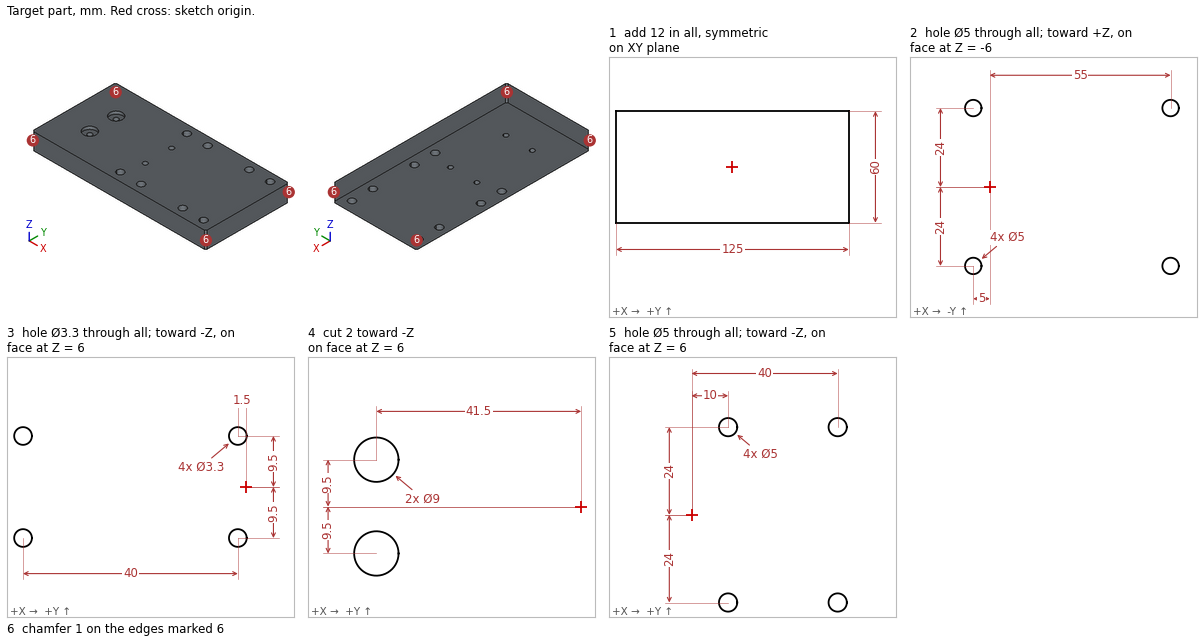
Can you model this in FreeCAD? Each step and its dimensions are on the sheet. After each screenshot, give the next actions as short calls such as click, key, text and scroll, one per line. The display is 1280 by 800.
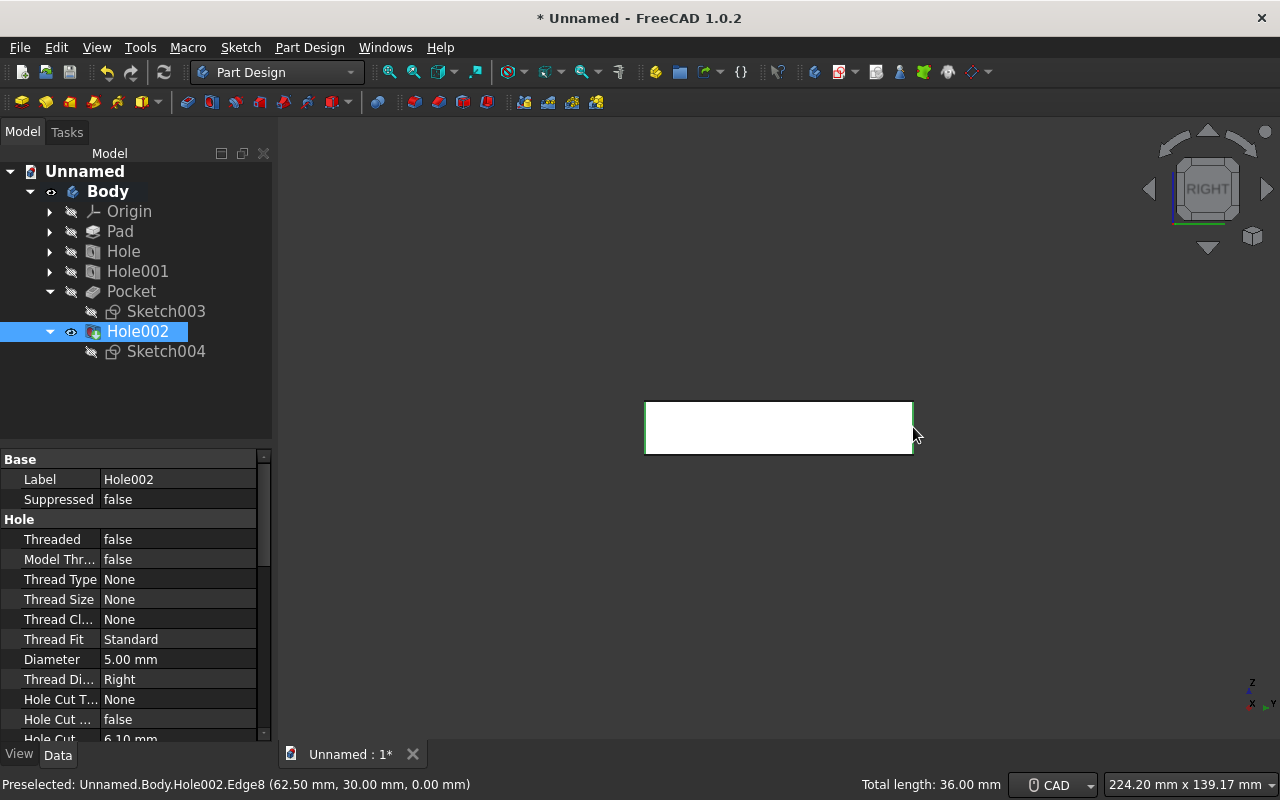
key(5)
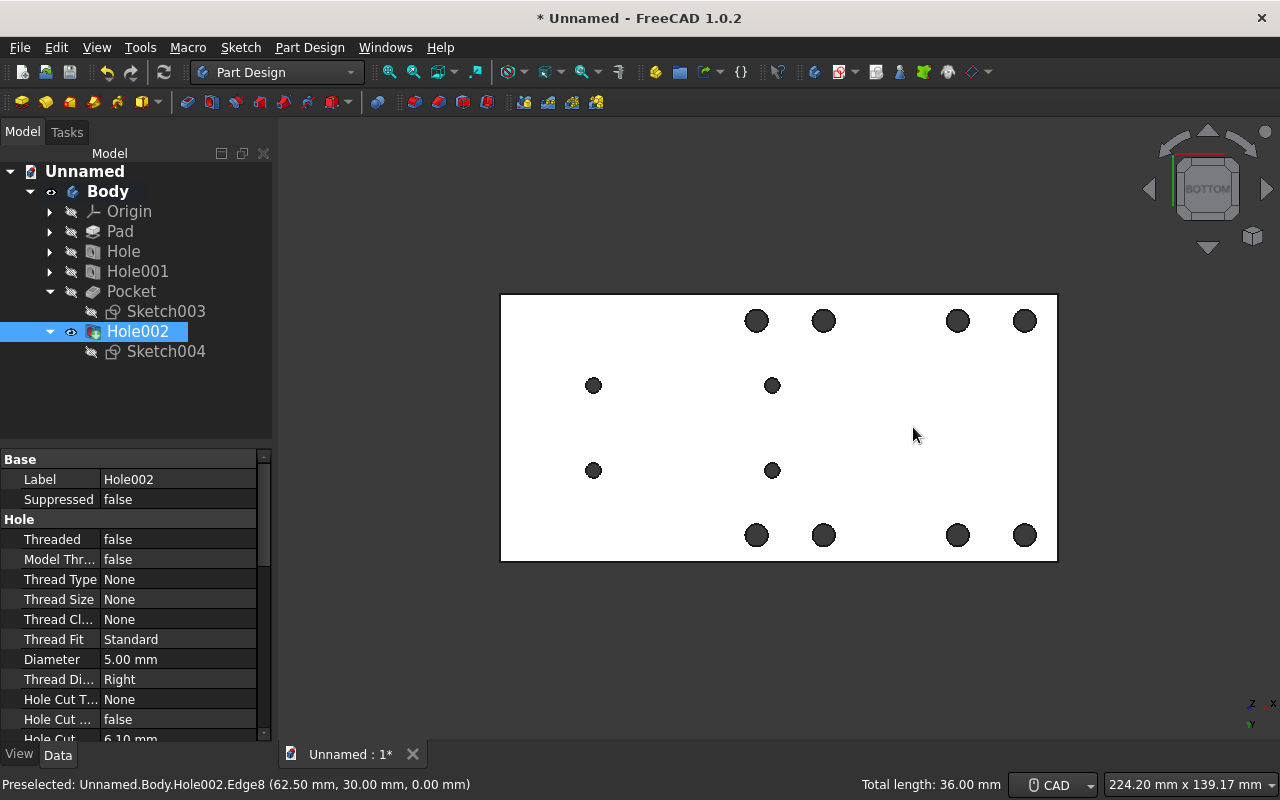
key(4)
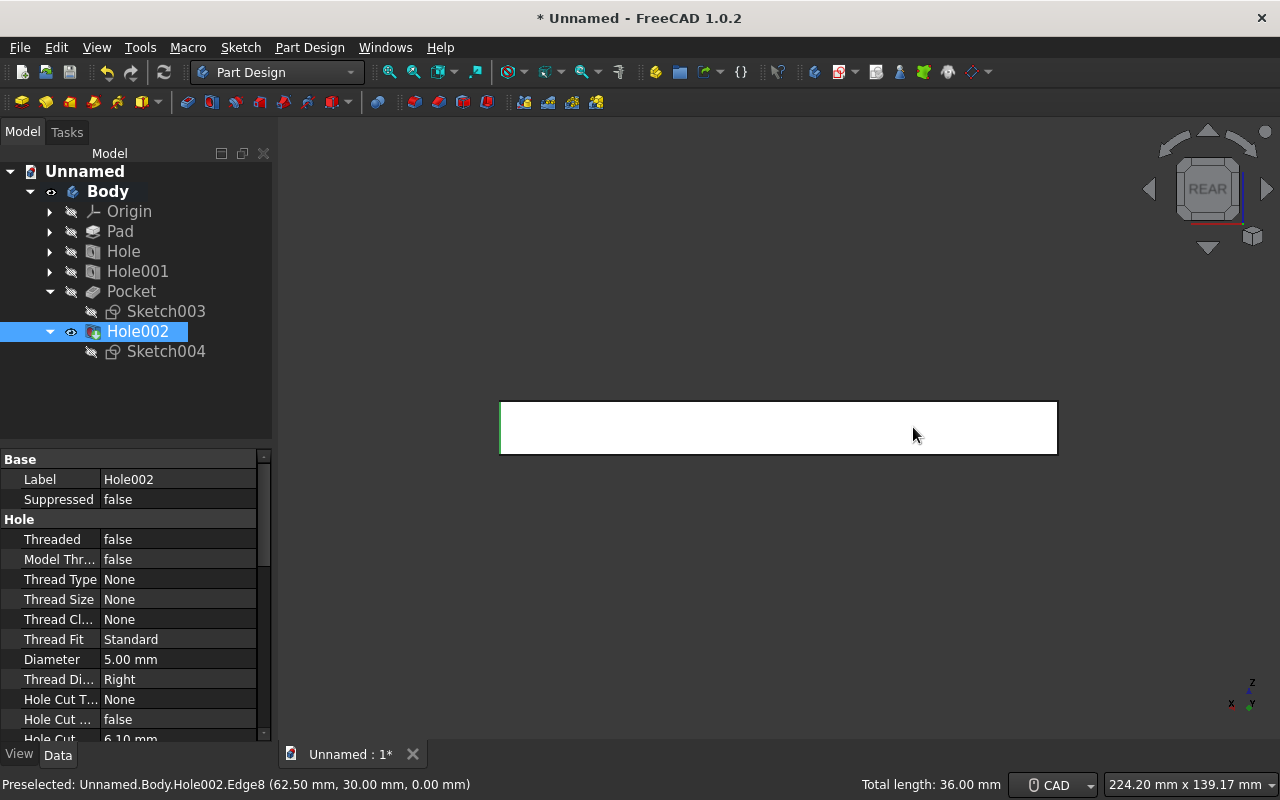
click(1058, 427, ctrl)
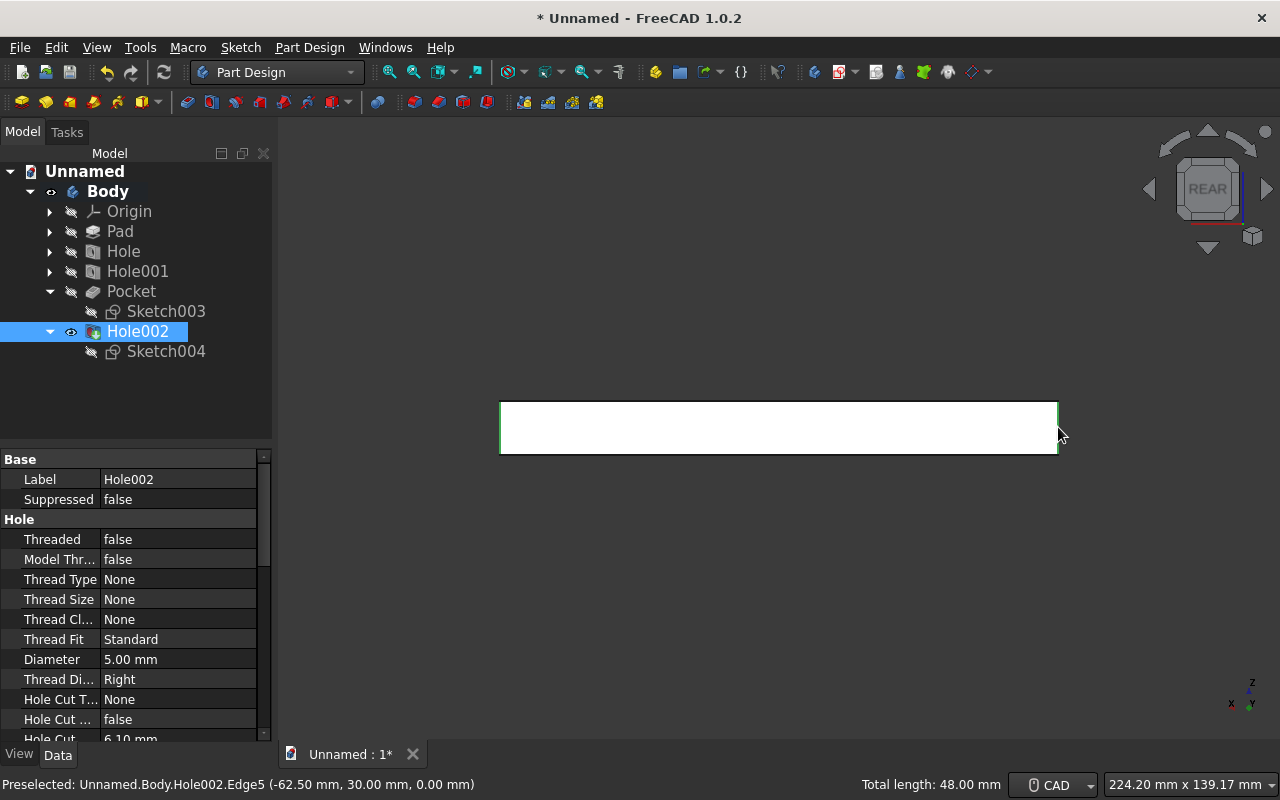
click(440, 102)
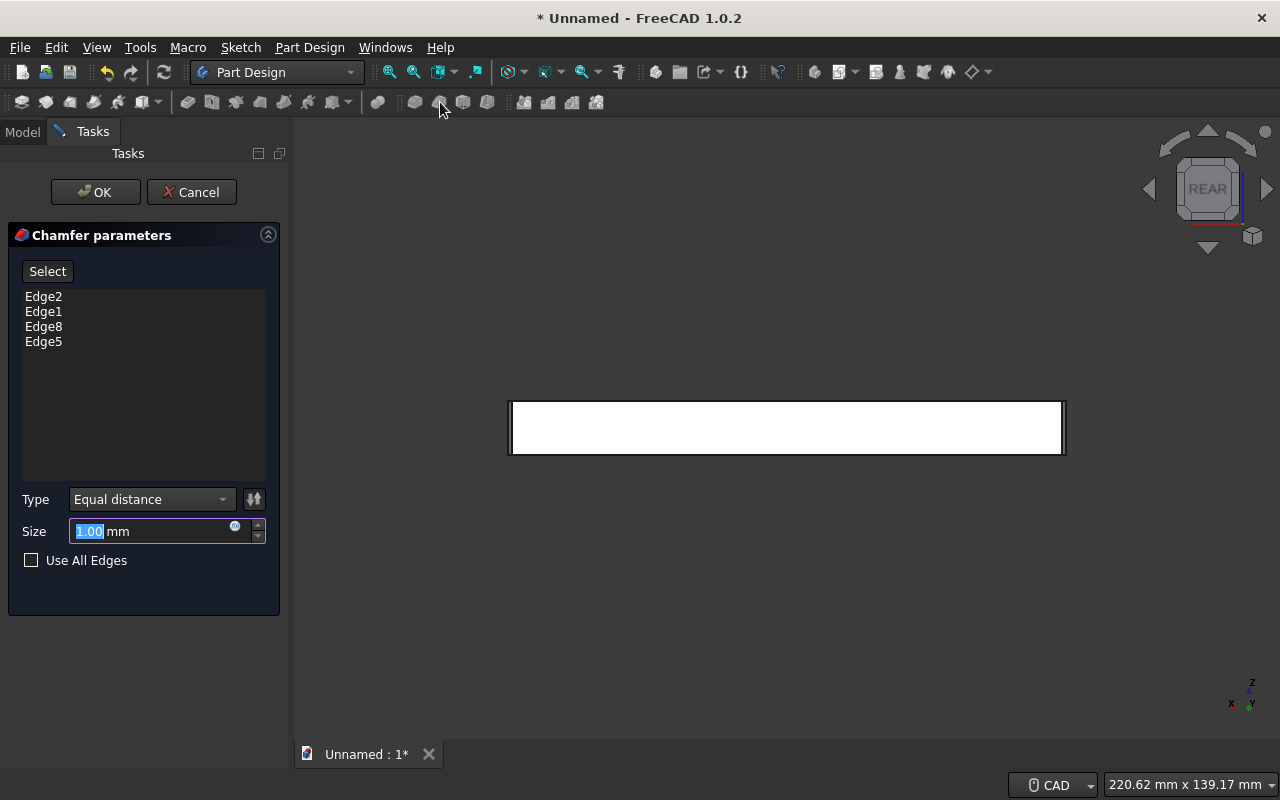
text(1)
key(Tab)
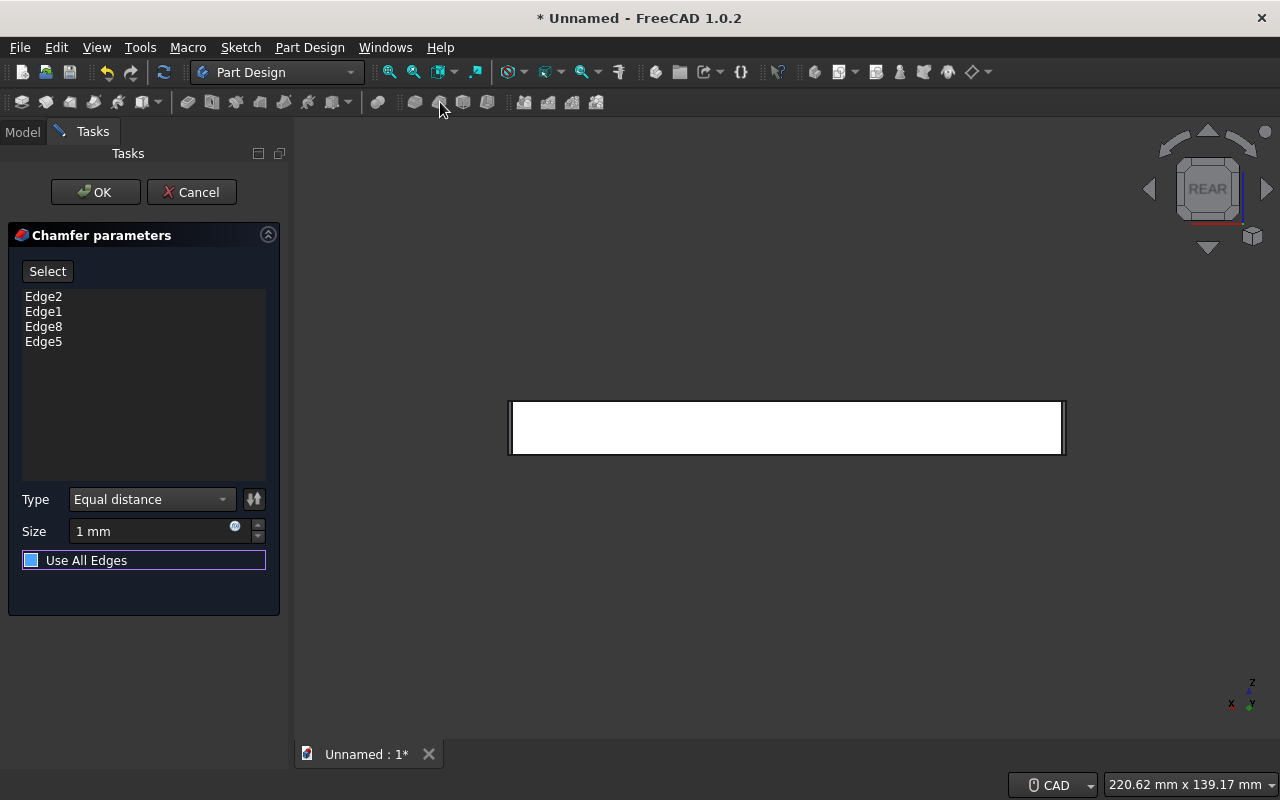
click(96, 192)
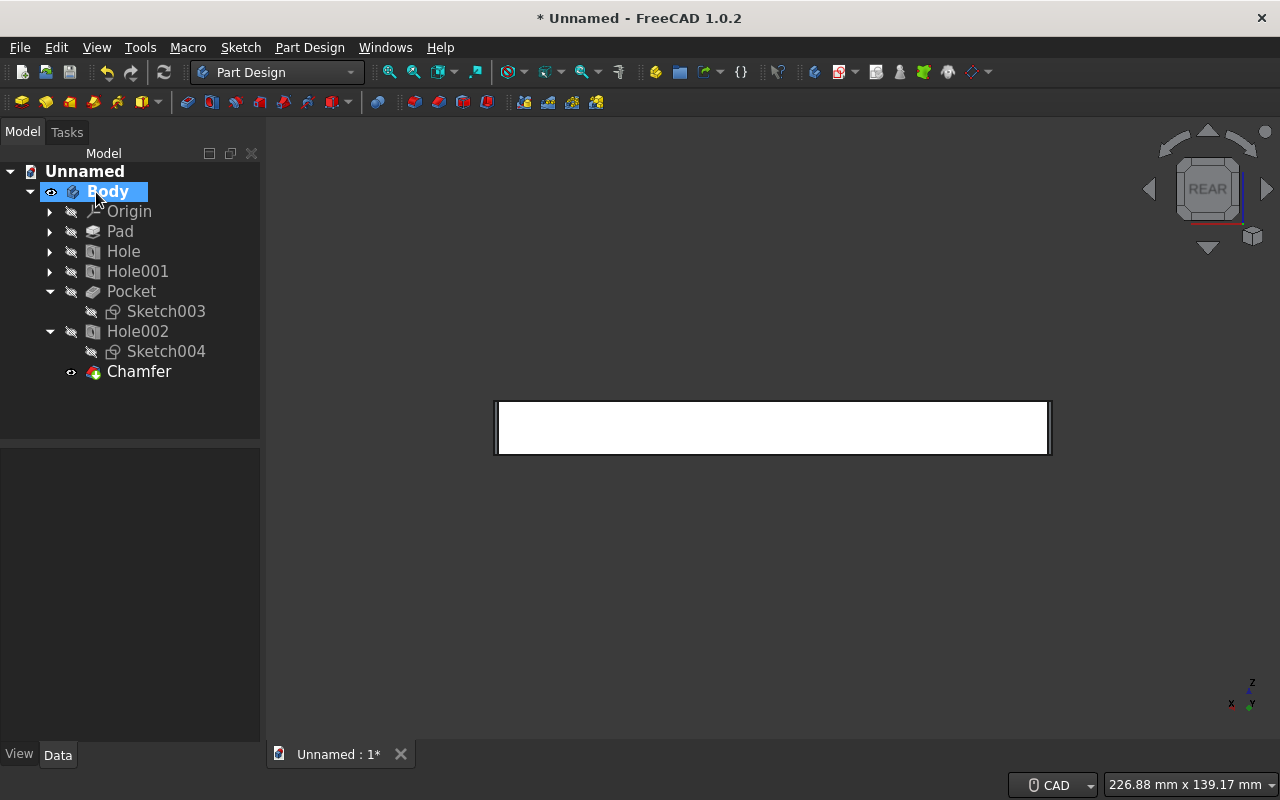
key(0)